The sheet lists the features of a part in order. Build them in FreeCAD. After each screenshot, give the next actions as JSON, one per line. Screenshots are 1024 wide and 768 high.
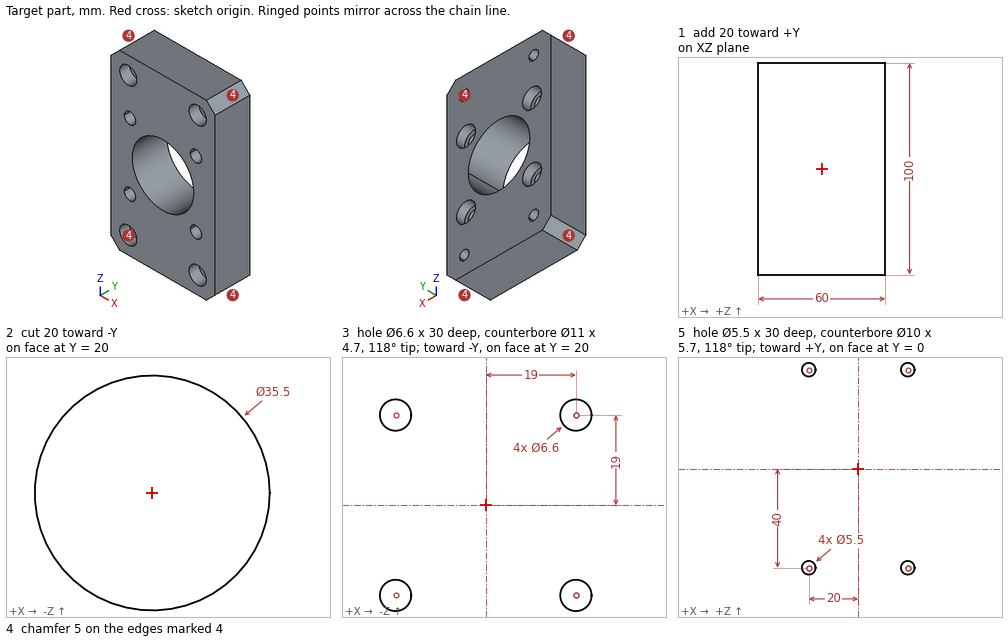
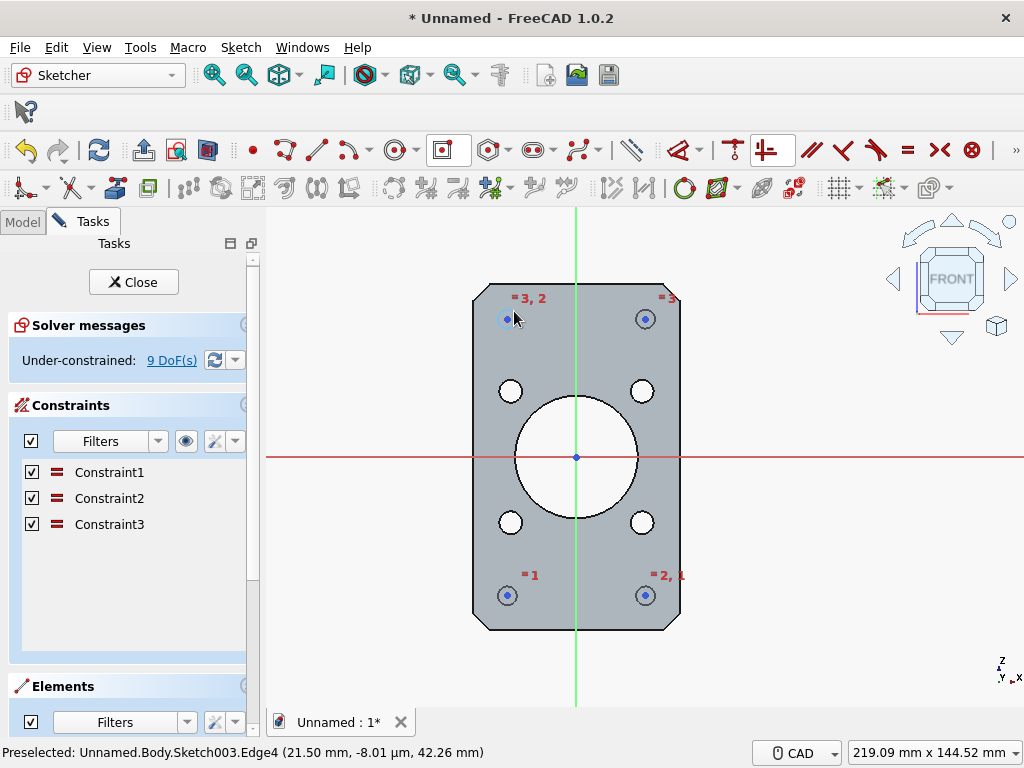
{"action": "left_click", "coordinate": [507, 596]}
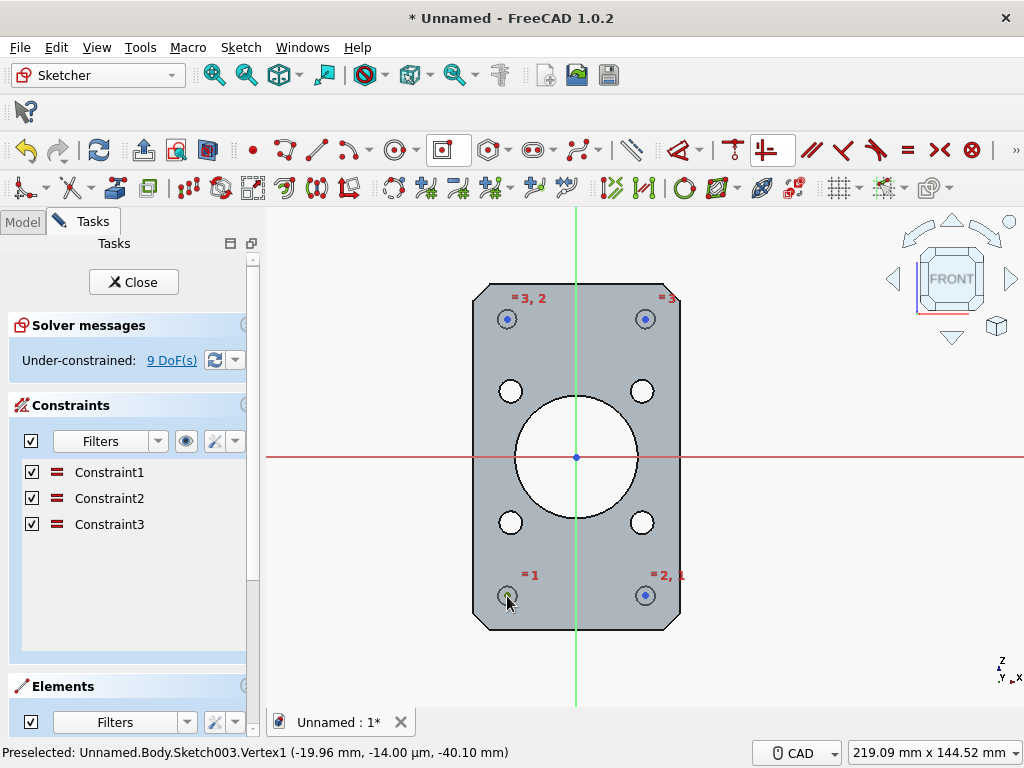
{"action": "left_click", "coordinate": [646, 596]}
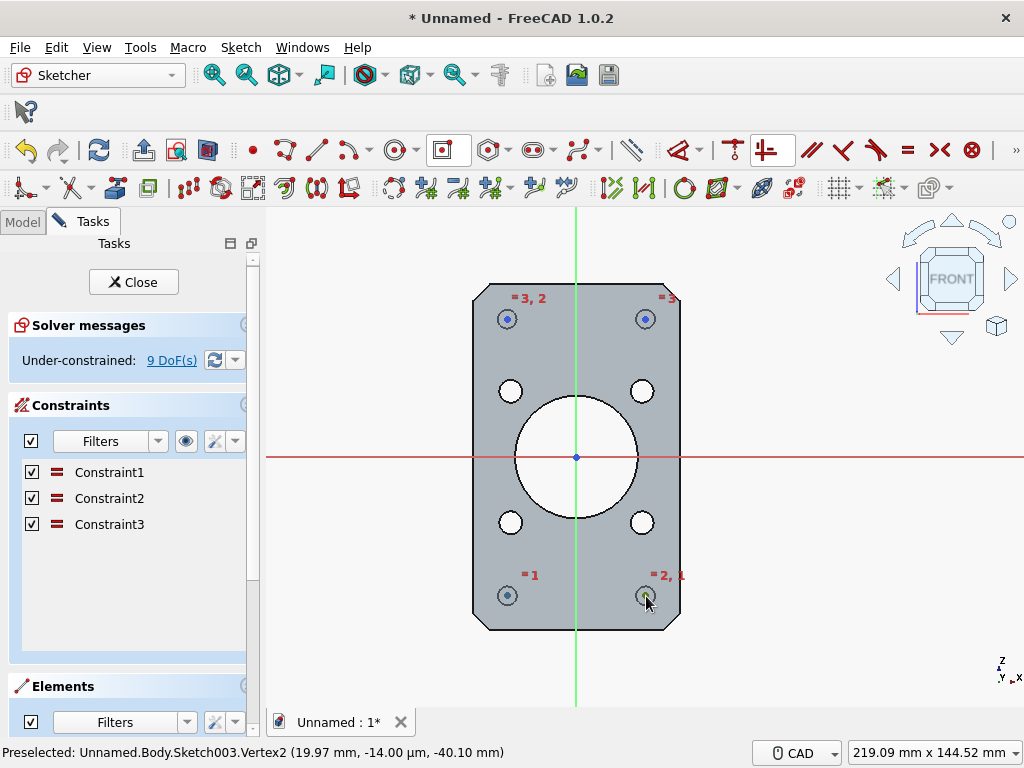
{"action": "left_click", "coordinate": [576, 647]}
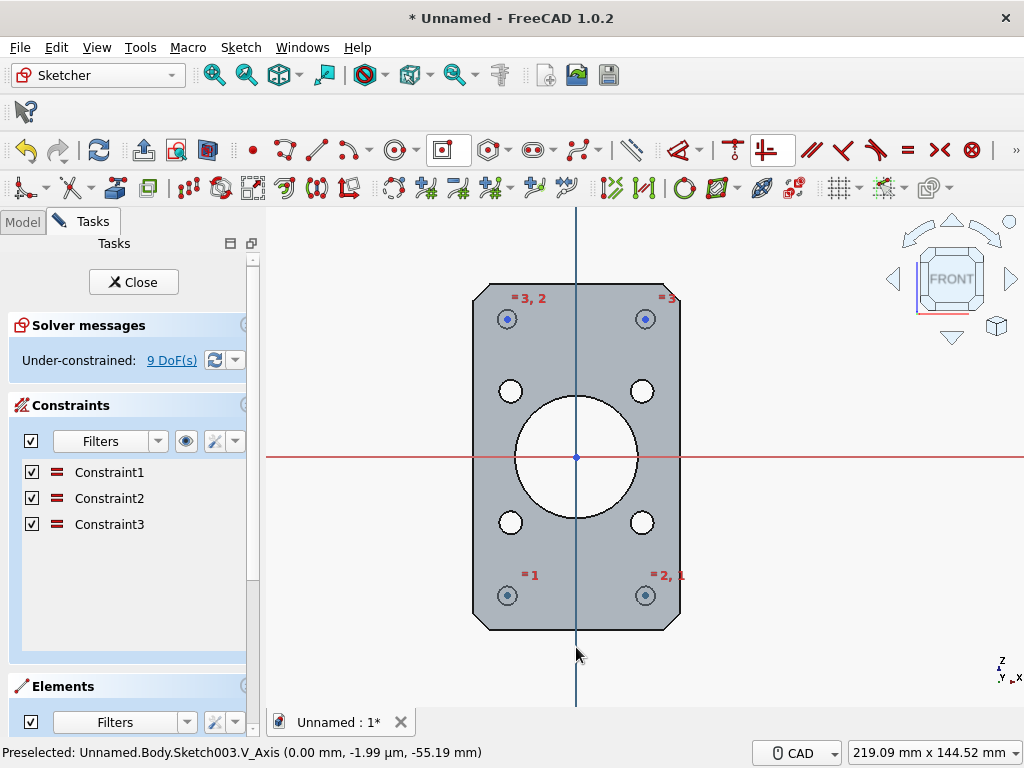
{"action": "key", "text": "s"}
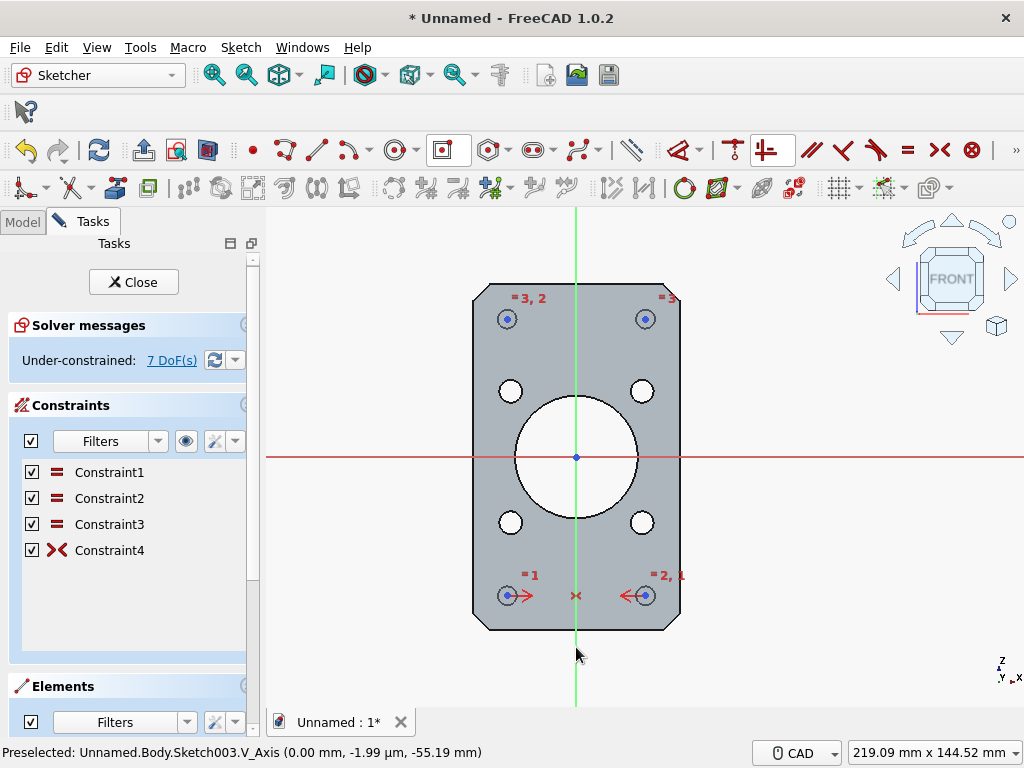
{"action": "left_click", "coordinate": [507, 596]}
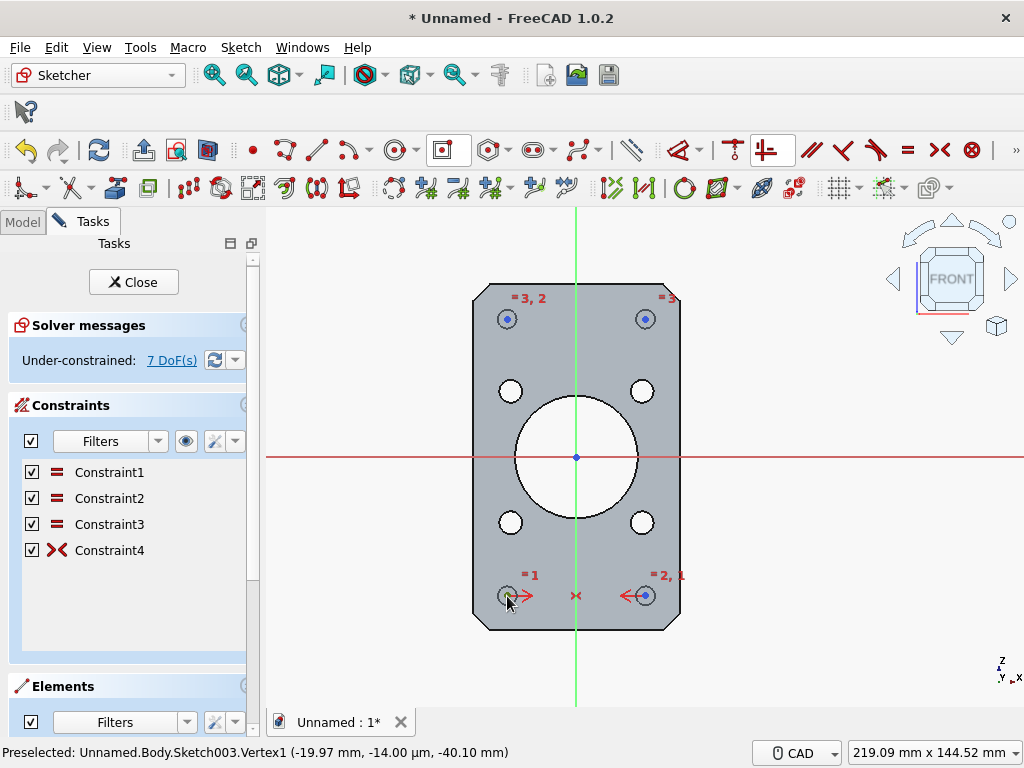
{"action": "left_click", "coordinate": [507, 319]}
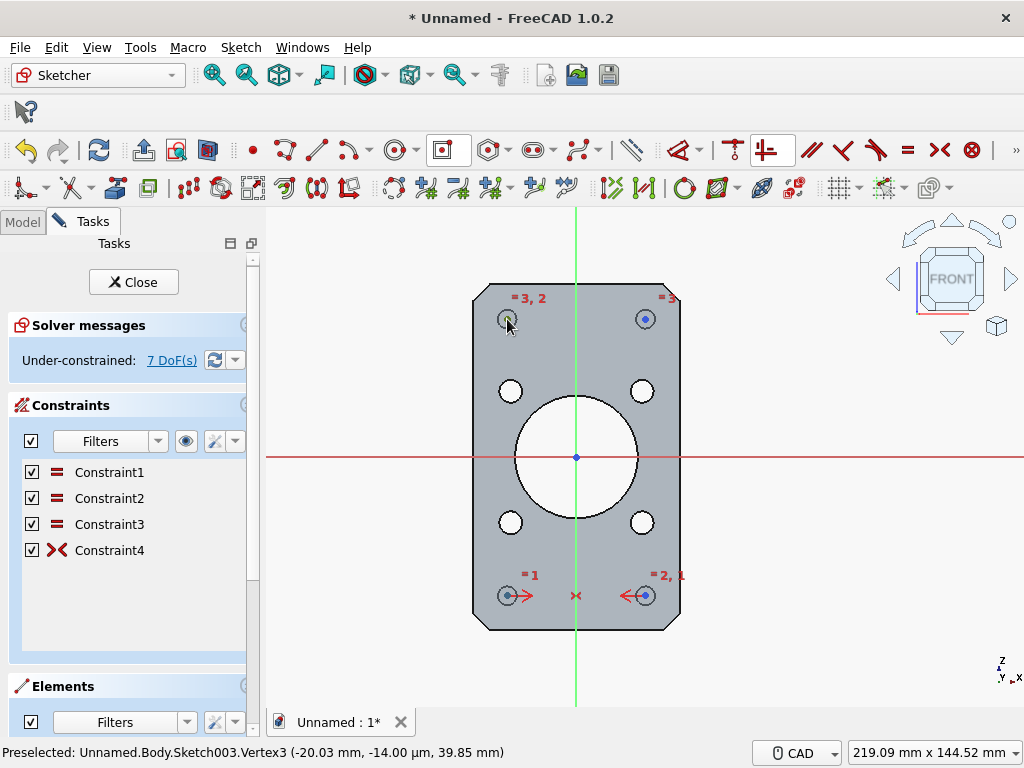
{"action": "left_click", "coordinate": [334, 457]}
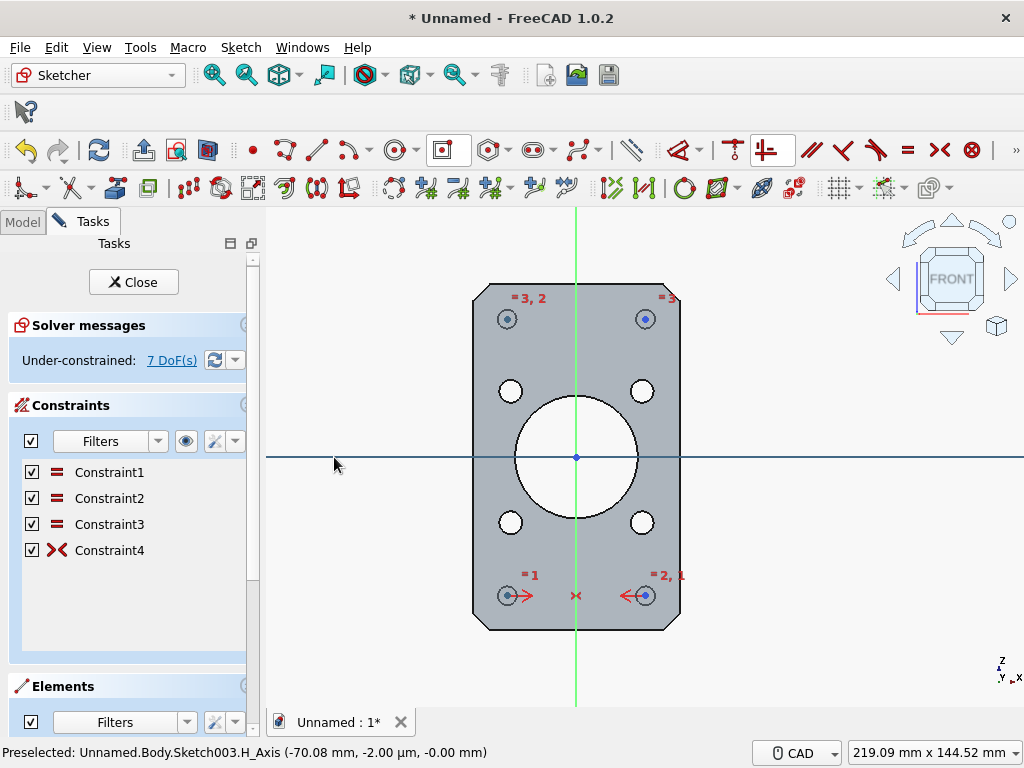
{"action": "left_click", "coordinate": [940, 150]}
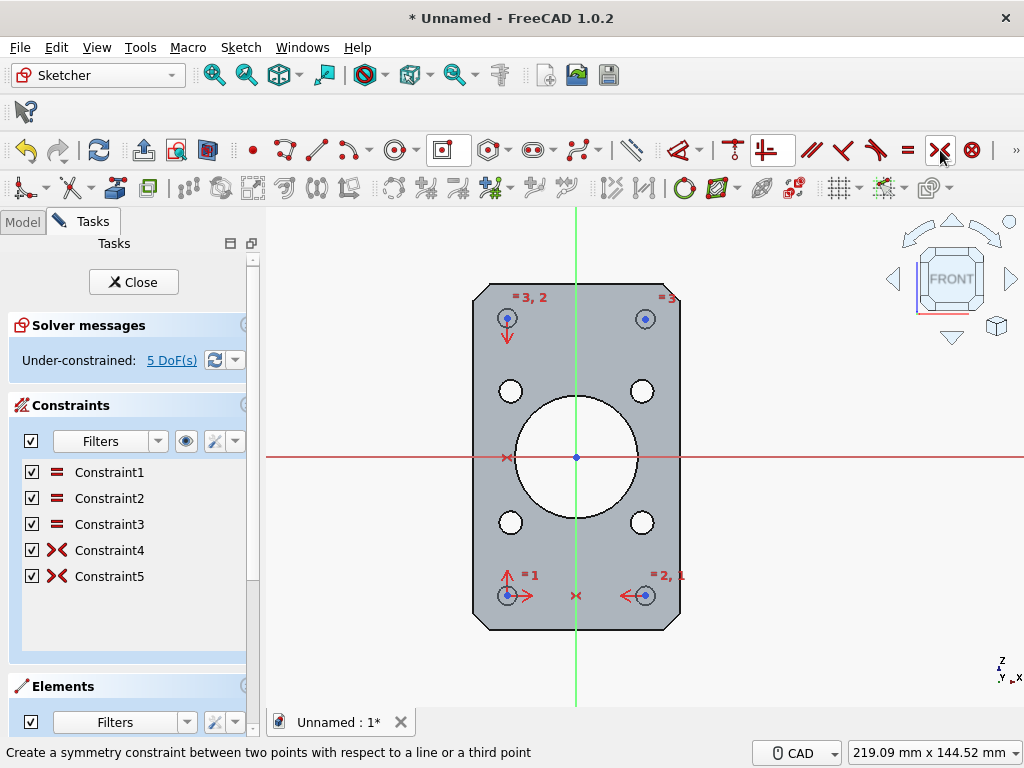
{"action": "left_click", "coordinate": [646, 596]}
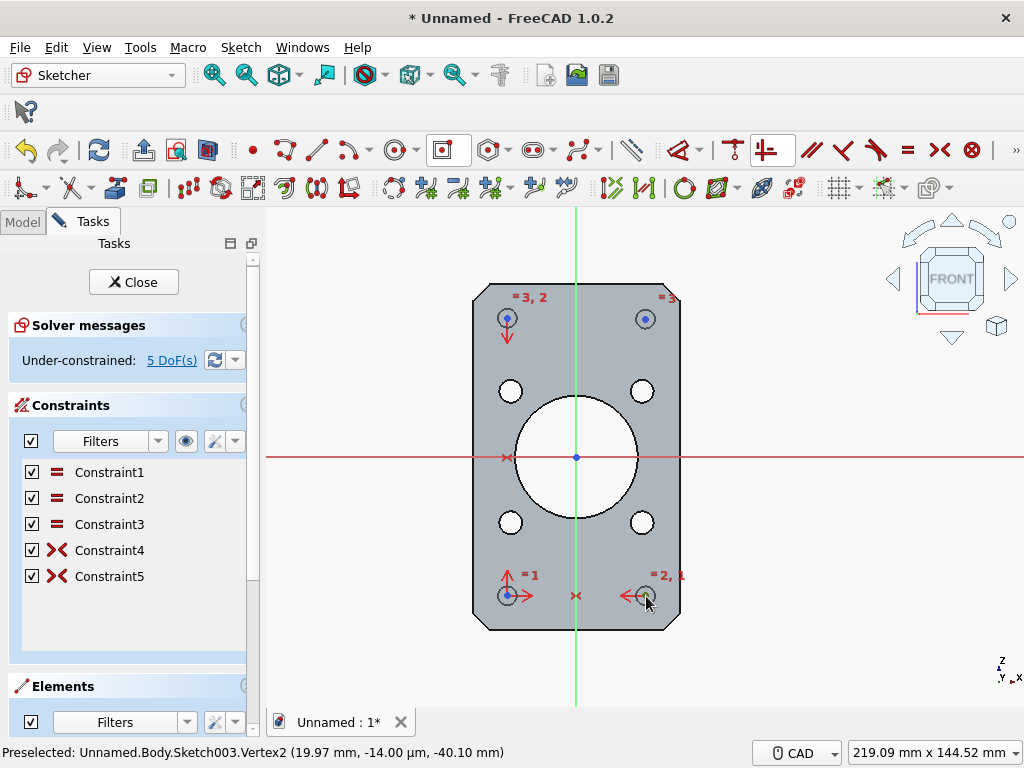
{"action": "left_click", "coordinate": [646, 319]}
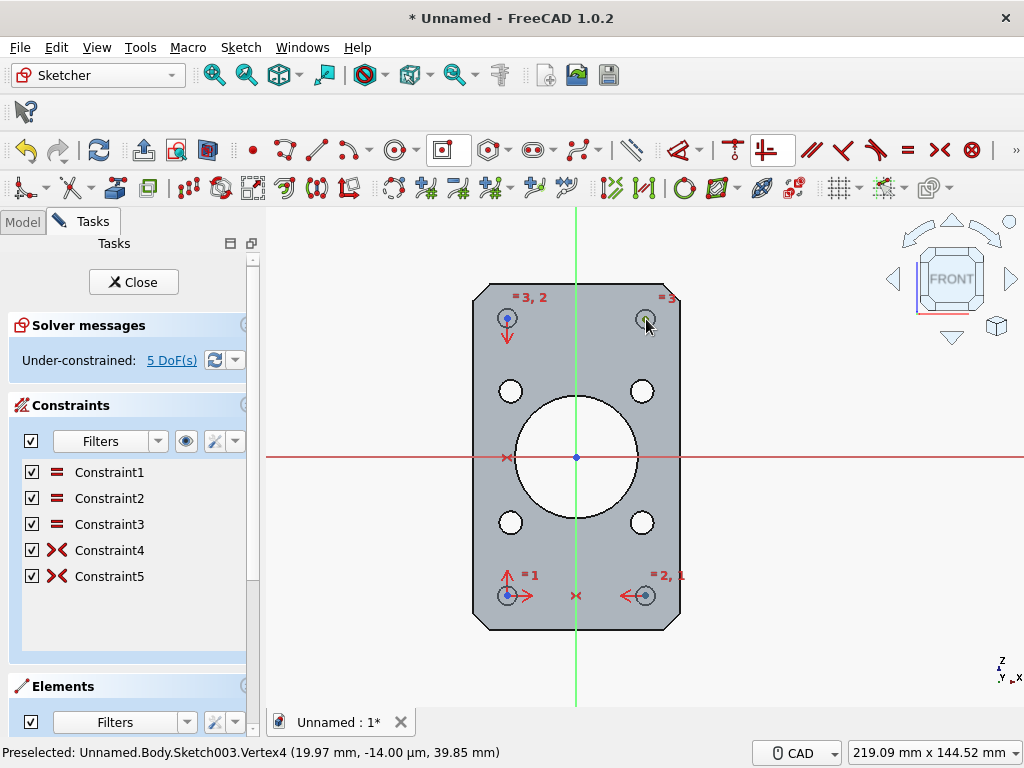
{"action": "left_click", "coordinate": [334, 457]}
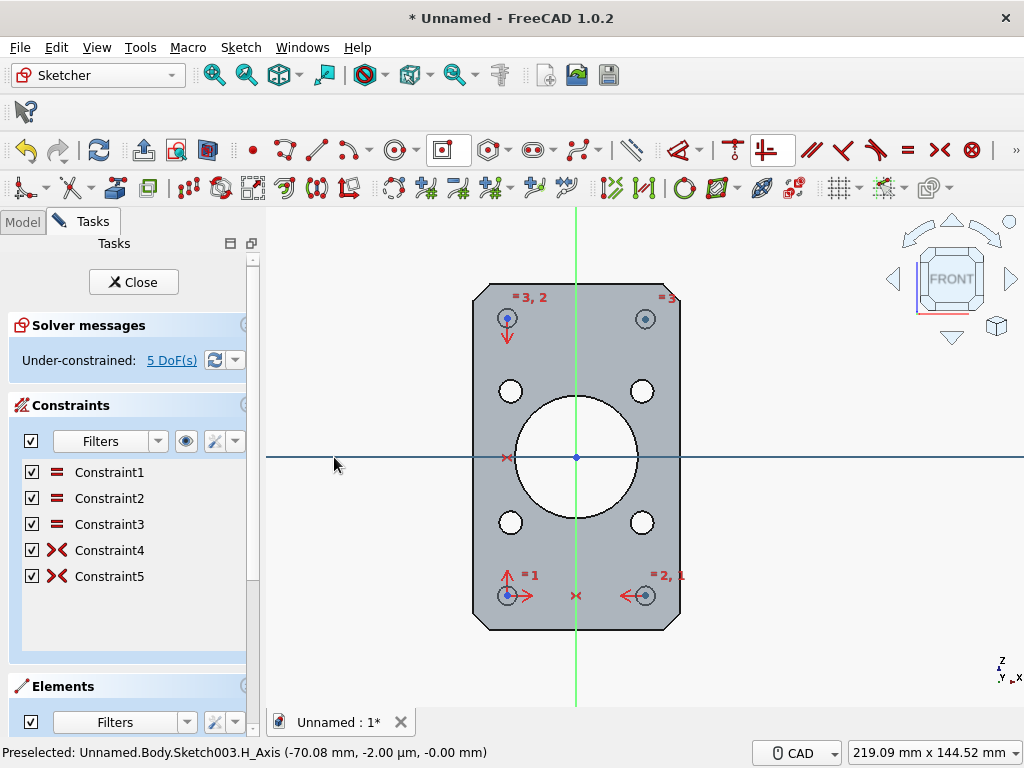
{"action": "left_click", "coordinate": [940, 150]}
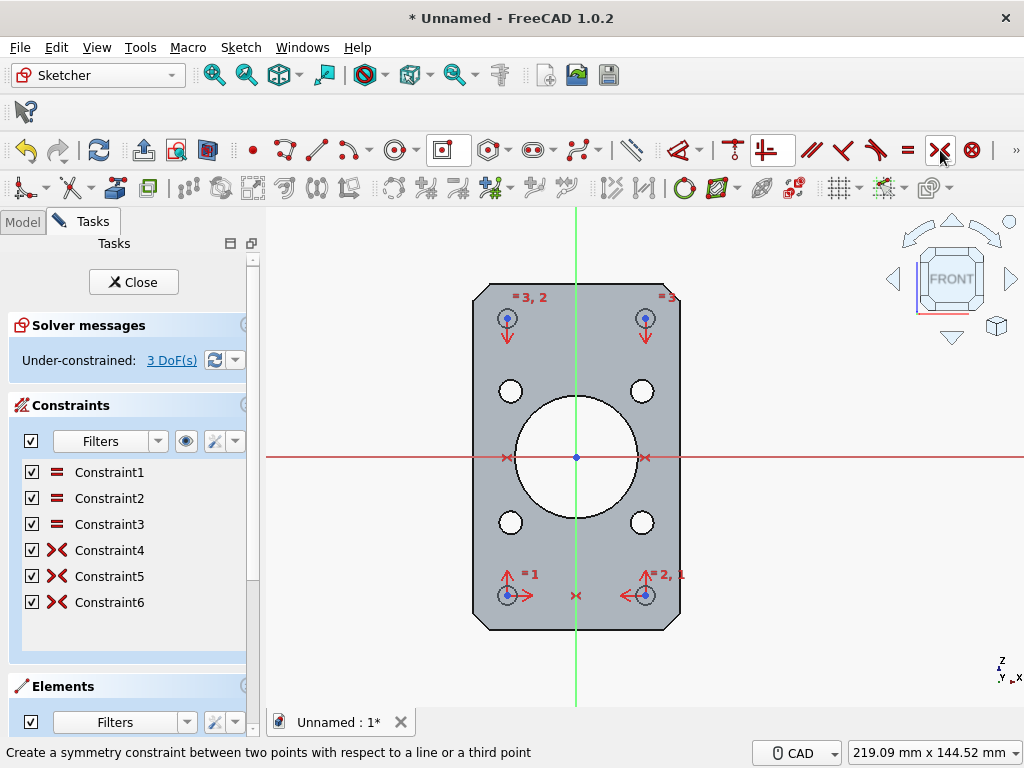
{"action": "left_click", "coordinate": [678, 150]}